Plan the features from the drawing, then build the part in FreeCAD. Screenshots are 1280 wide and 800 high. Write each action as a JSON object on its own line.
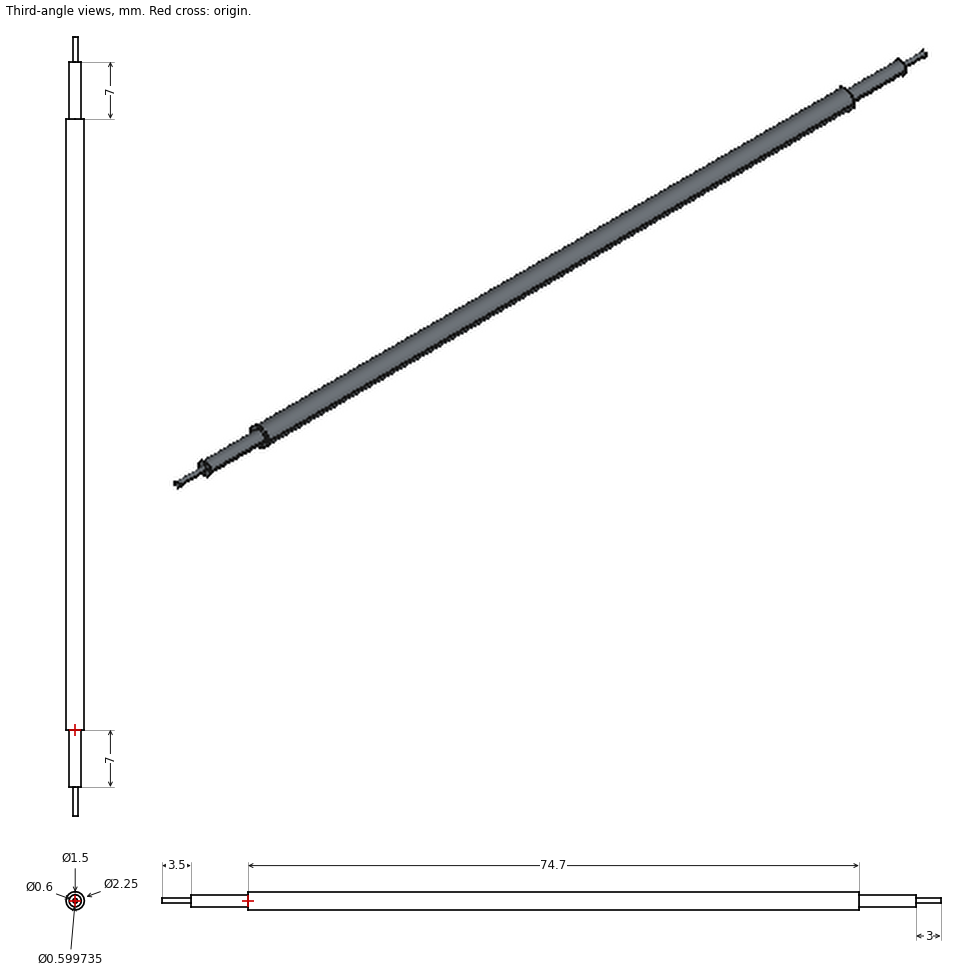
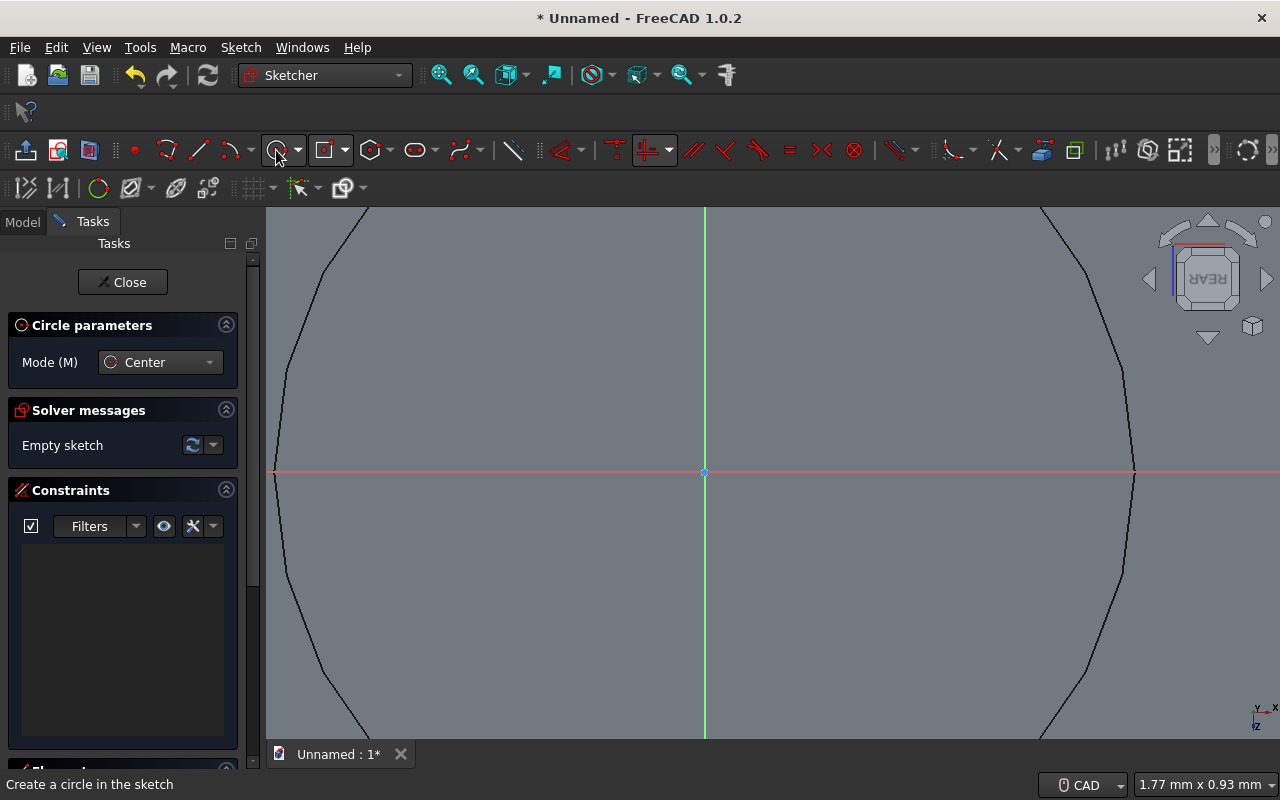
{"action": "left_click", "coordinate": [705, 472]}
{"action": "mouse_move", "coordinate": [826, 351]}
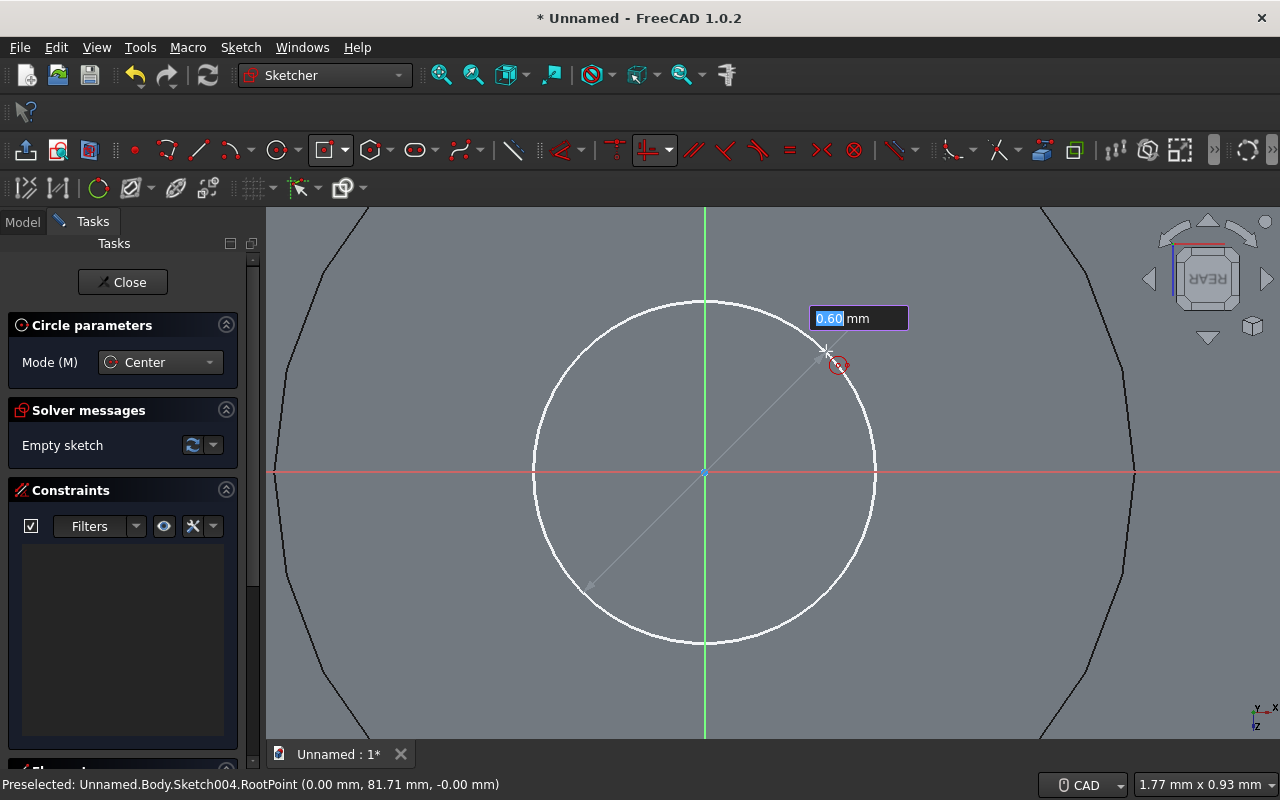
{"action": "type", "text": "0.599735"}
{"action": "key", "text": "Return"}
{"action": "key", "text": "Escape"}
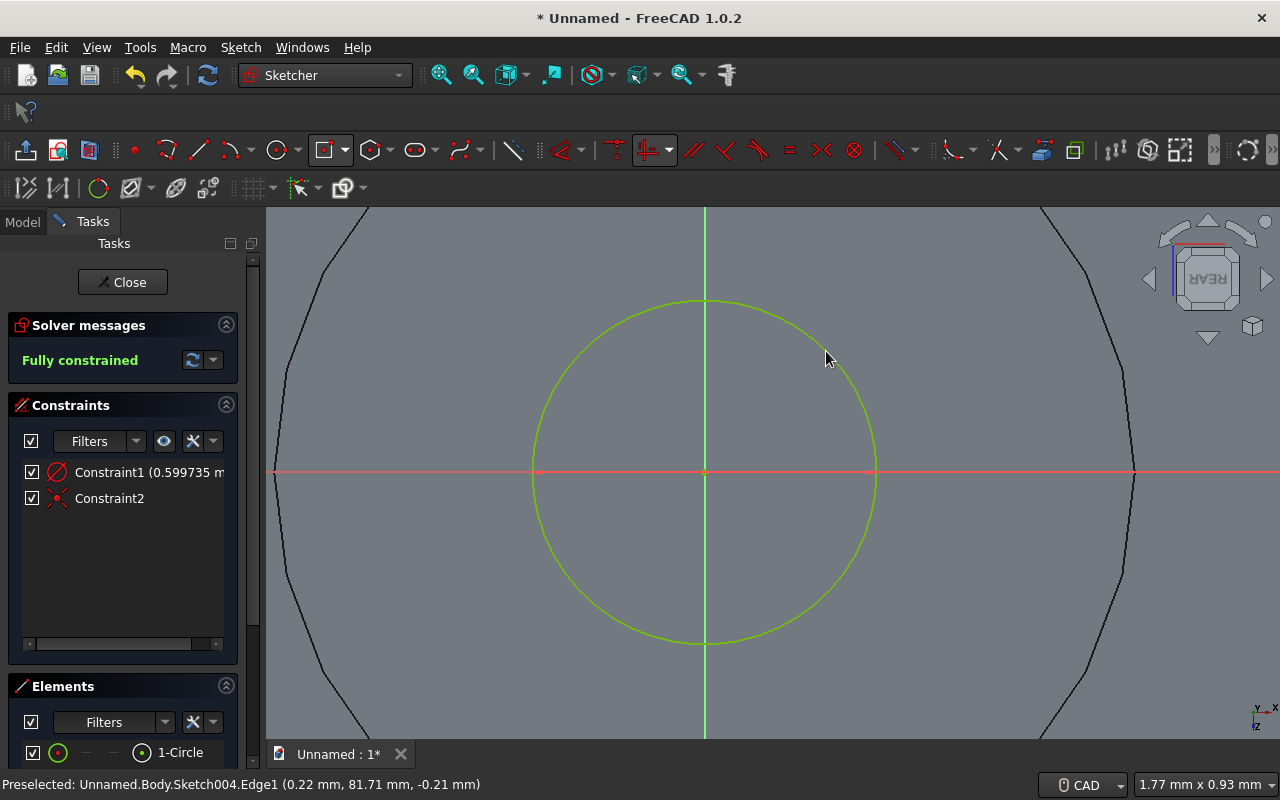
{"action": "left_click", "coordinate": [123, 282]}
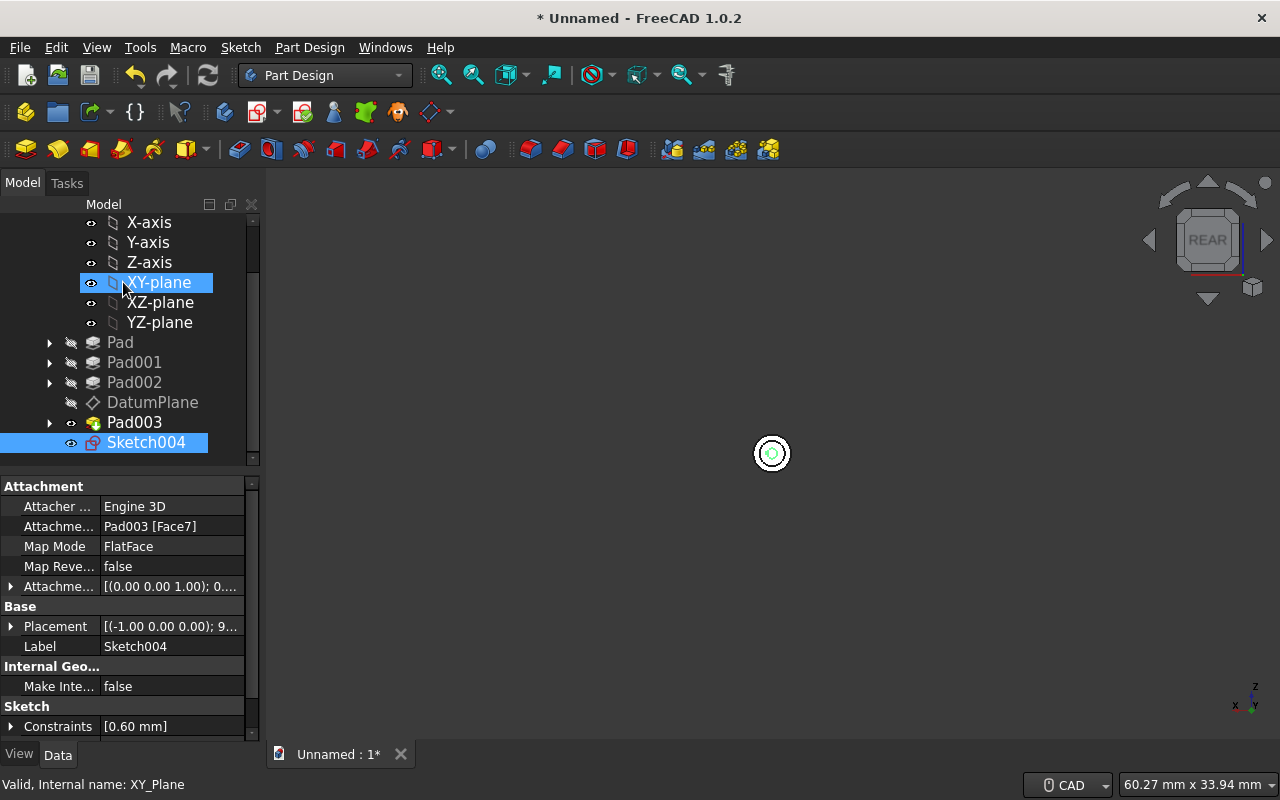
{"action": "left_click", "coordinate": [26, 150]}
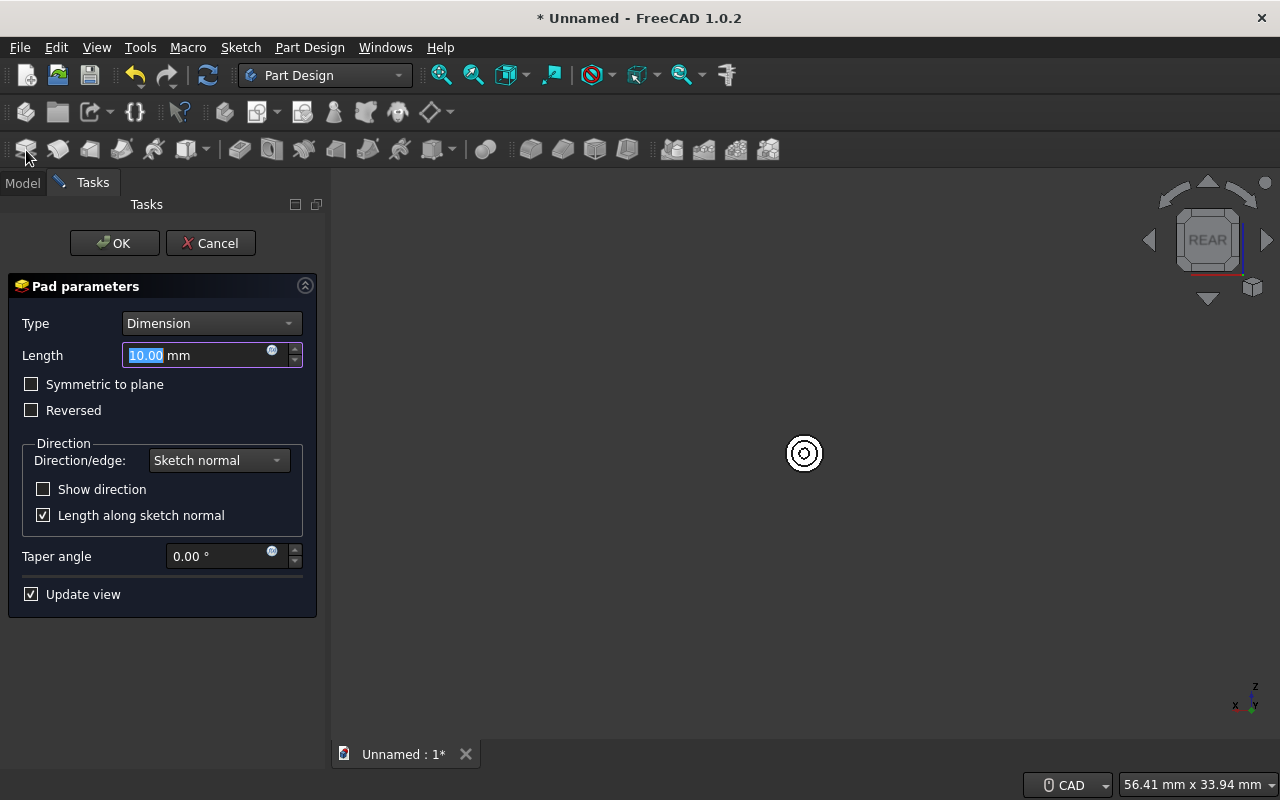
{"action": "type", "text": "3"}
{"action": "key", "text": "Tab"}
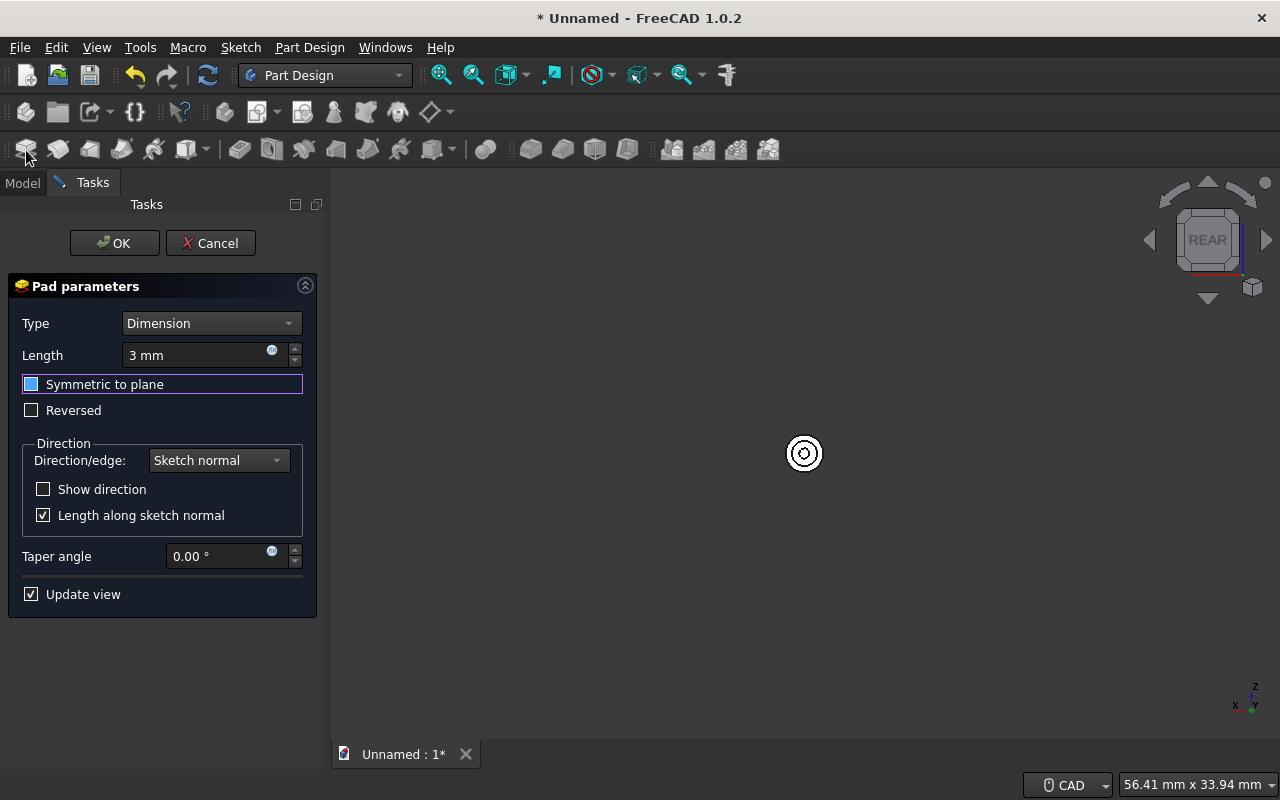
{"action": "left_click", "coordinate": [115, 243]}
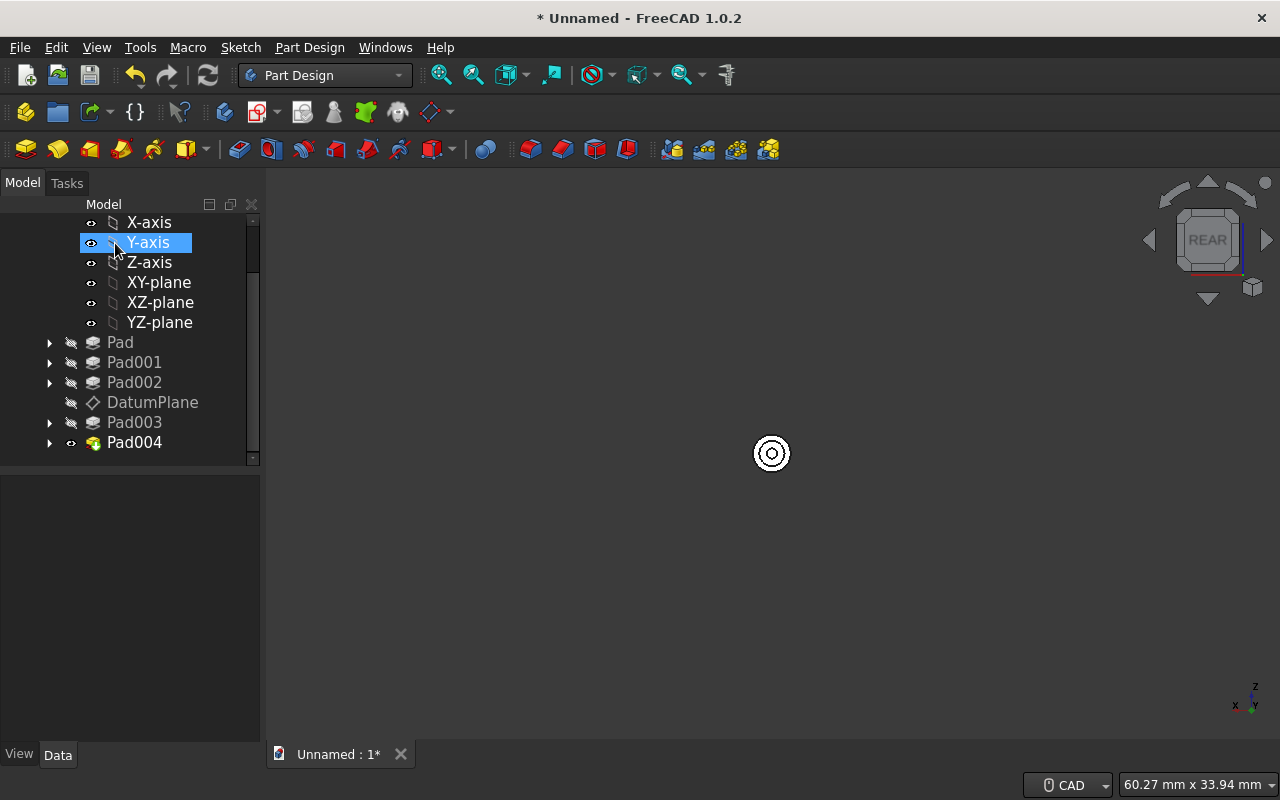
{"action": "key", "text": "0"}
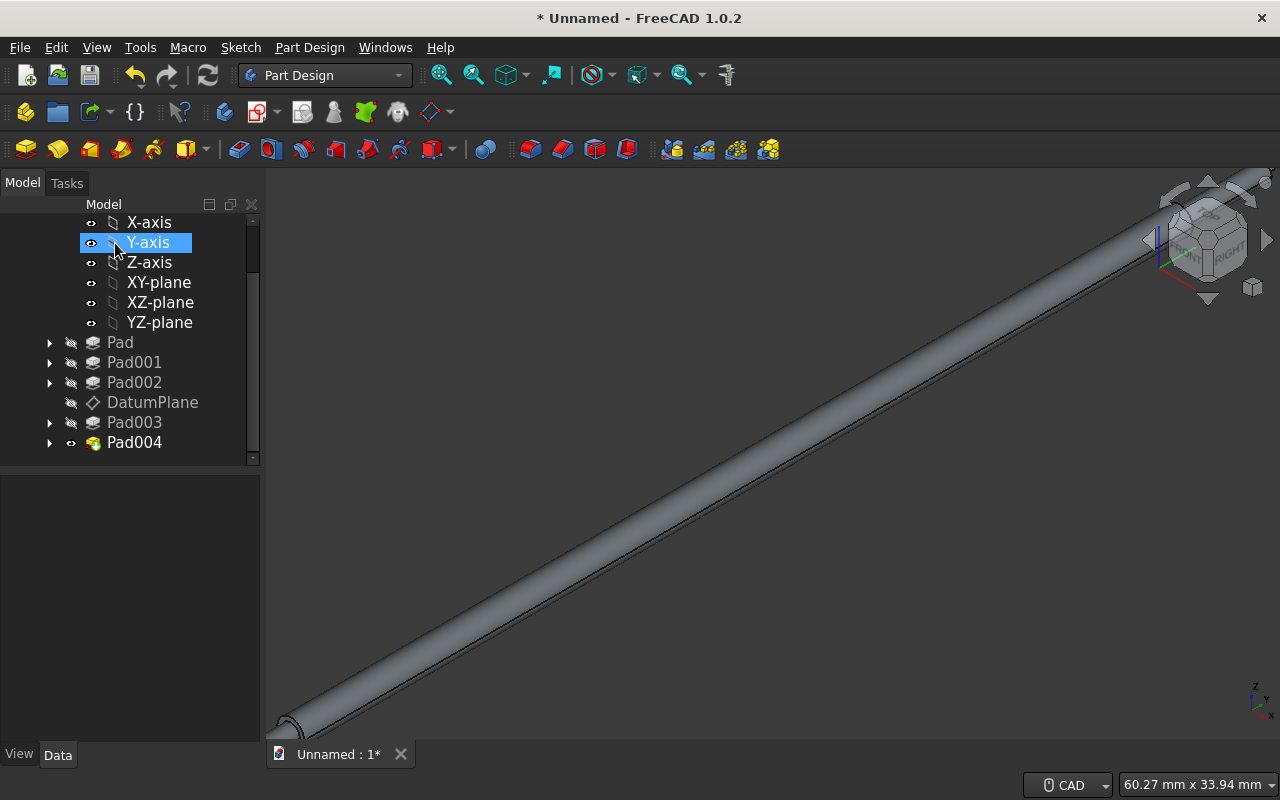
{"action": "left_click", "coordinate": [442, 76]}